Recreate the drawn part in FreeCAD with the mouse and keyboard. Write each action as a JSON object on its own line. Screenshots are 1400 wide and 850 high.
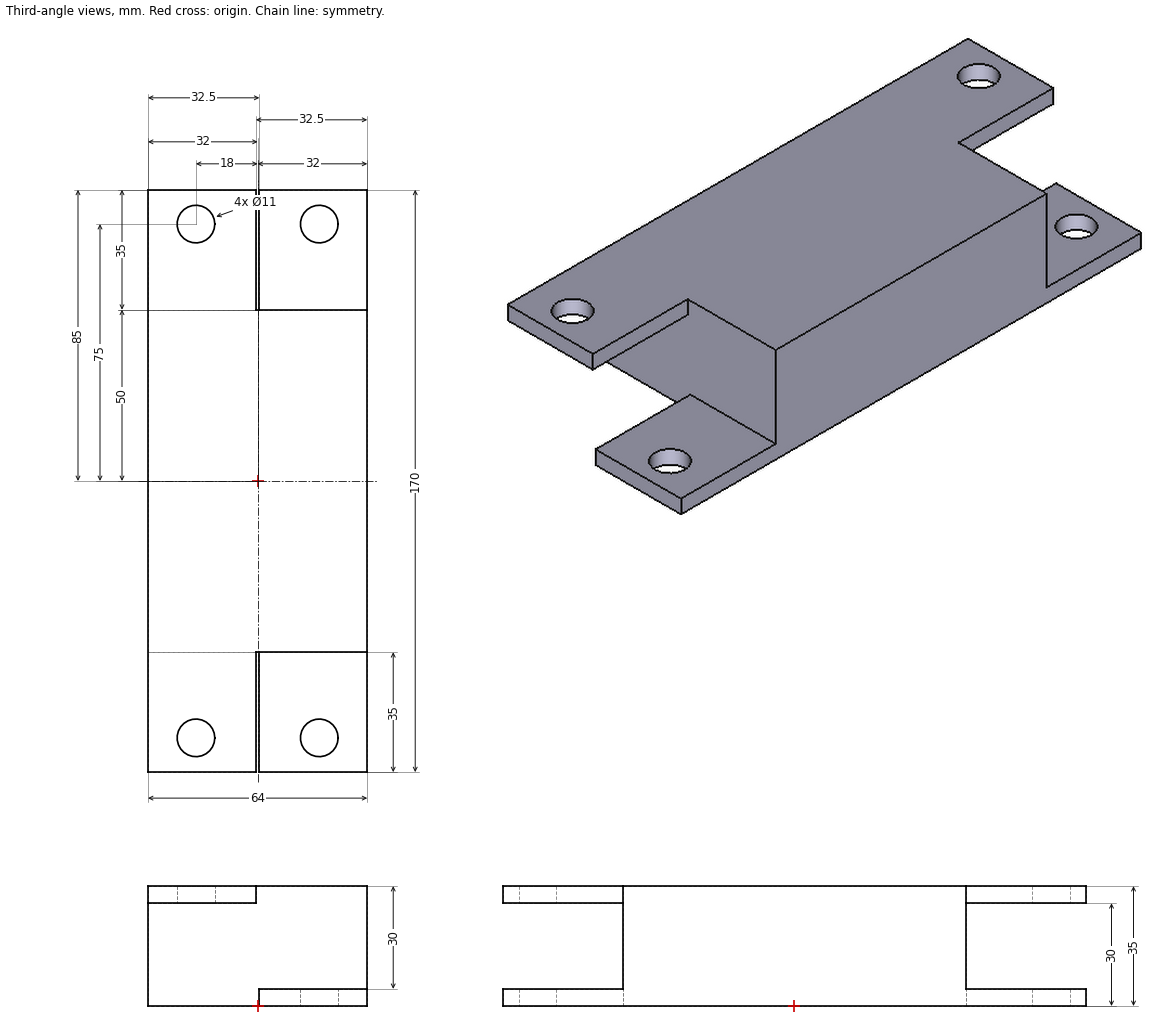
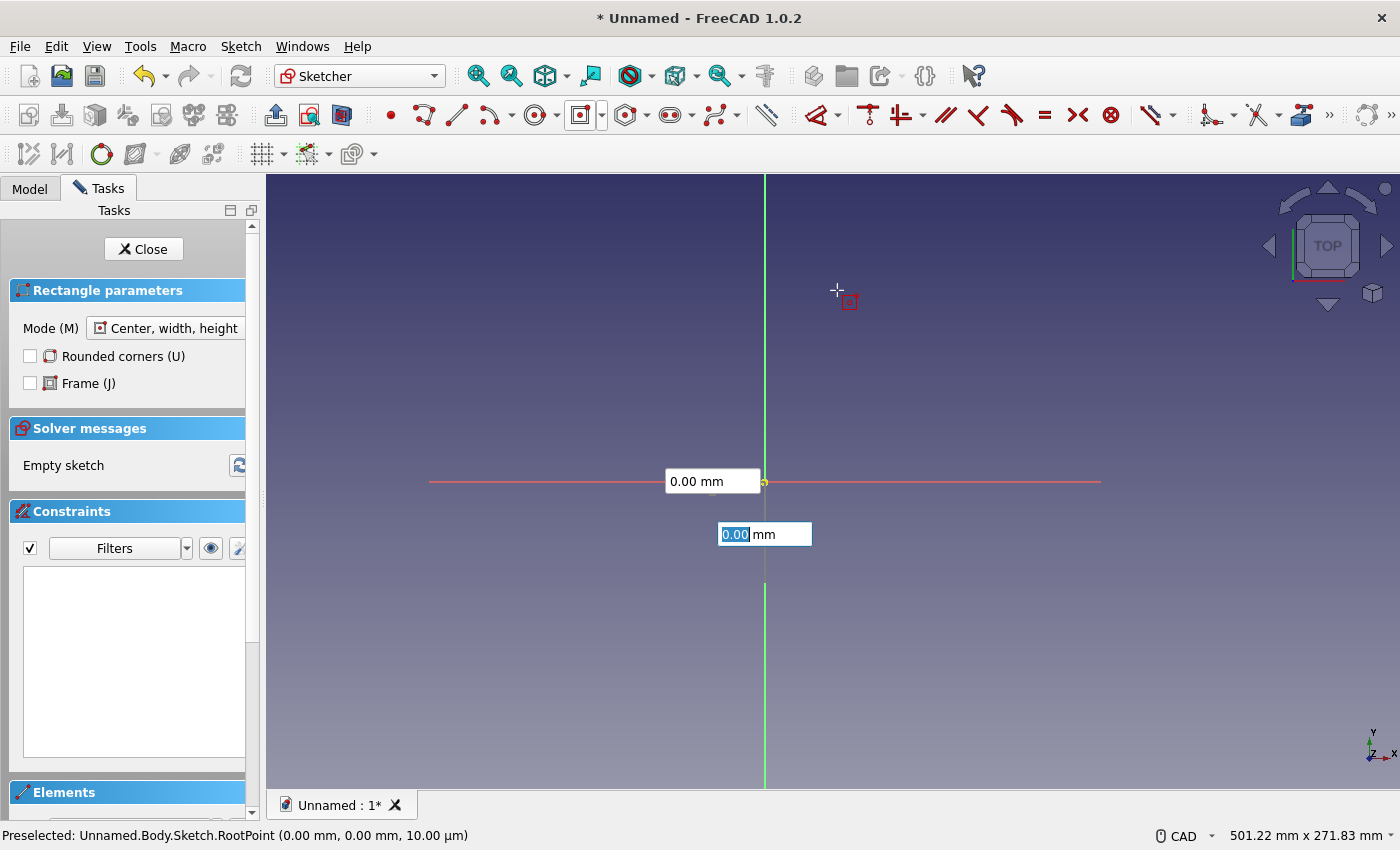
{"action": "type", "text": "64"}
{"action": "key", "text": "Tab"}
{"action": "type", "text": "170"}
{"action": "key", "text": "Return"}
{"action": "key", "text": "Escape"}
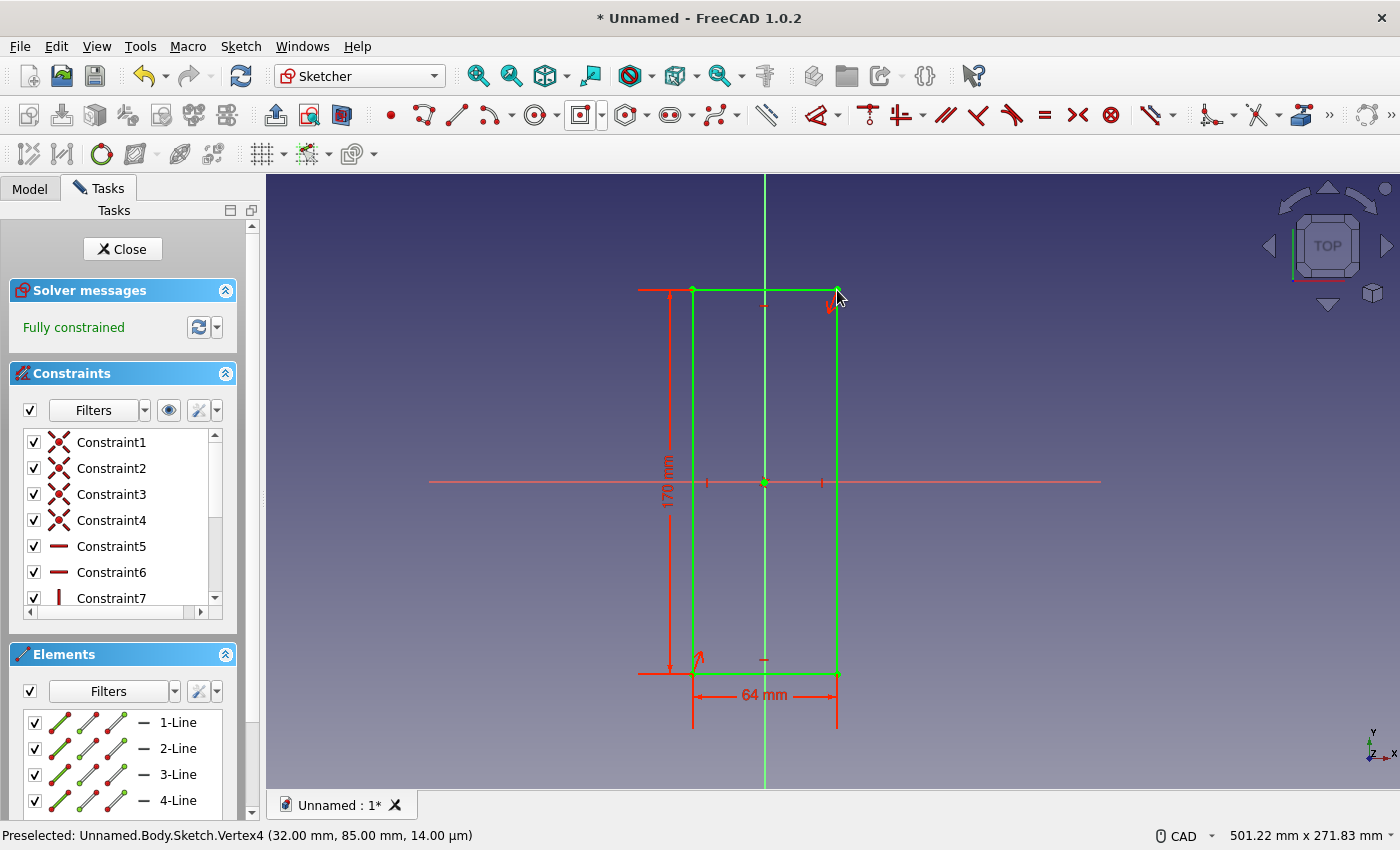
{"action": "left_click", "coordinate": [123, 249]}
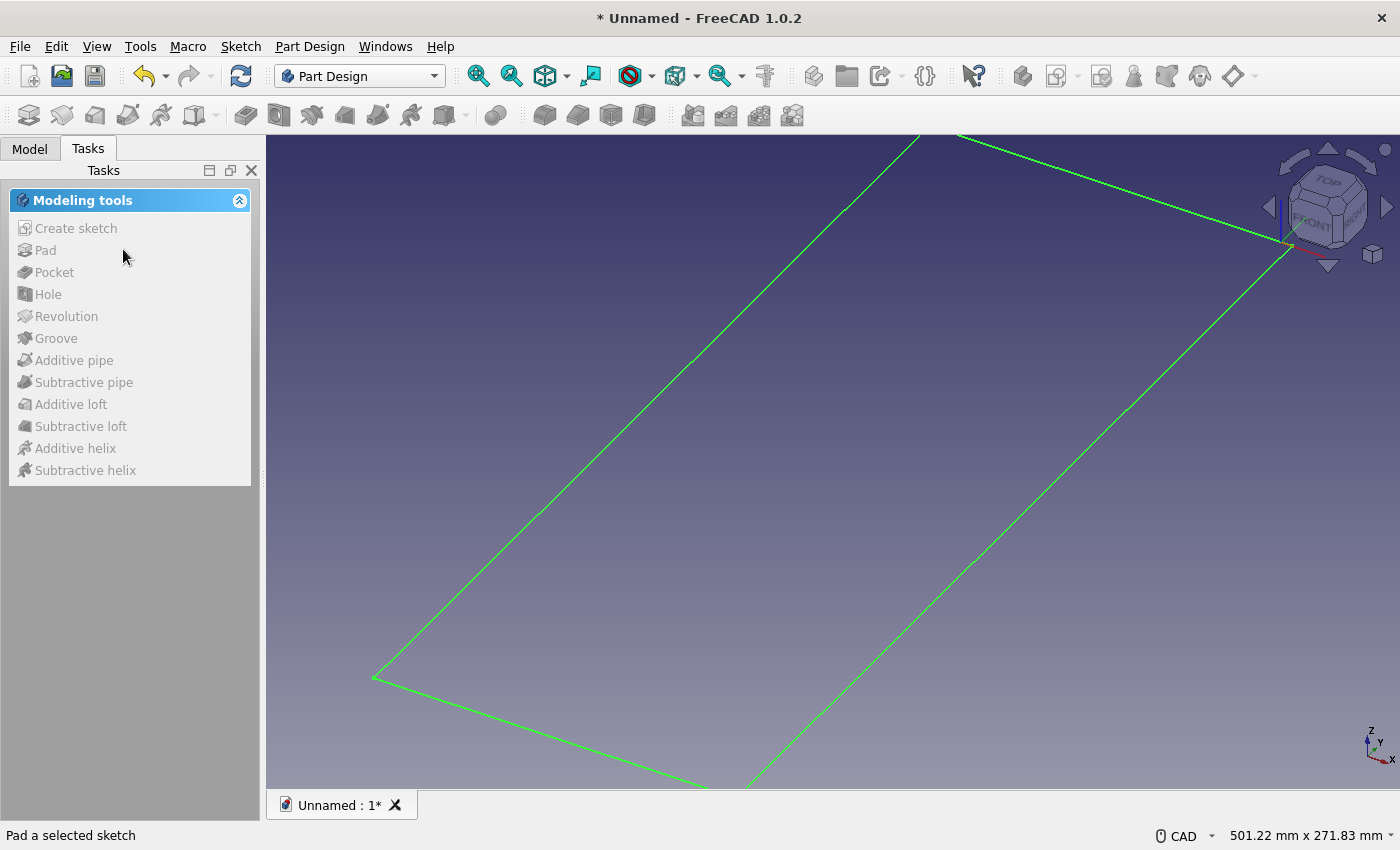
{"action": "left_click", "coordinate": [29, 116]}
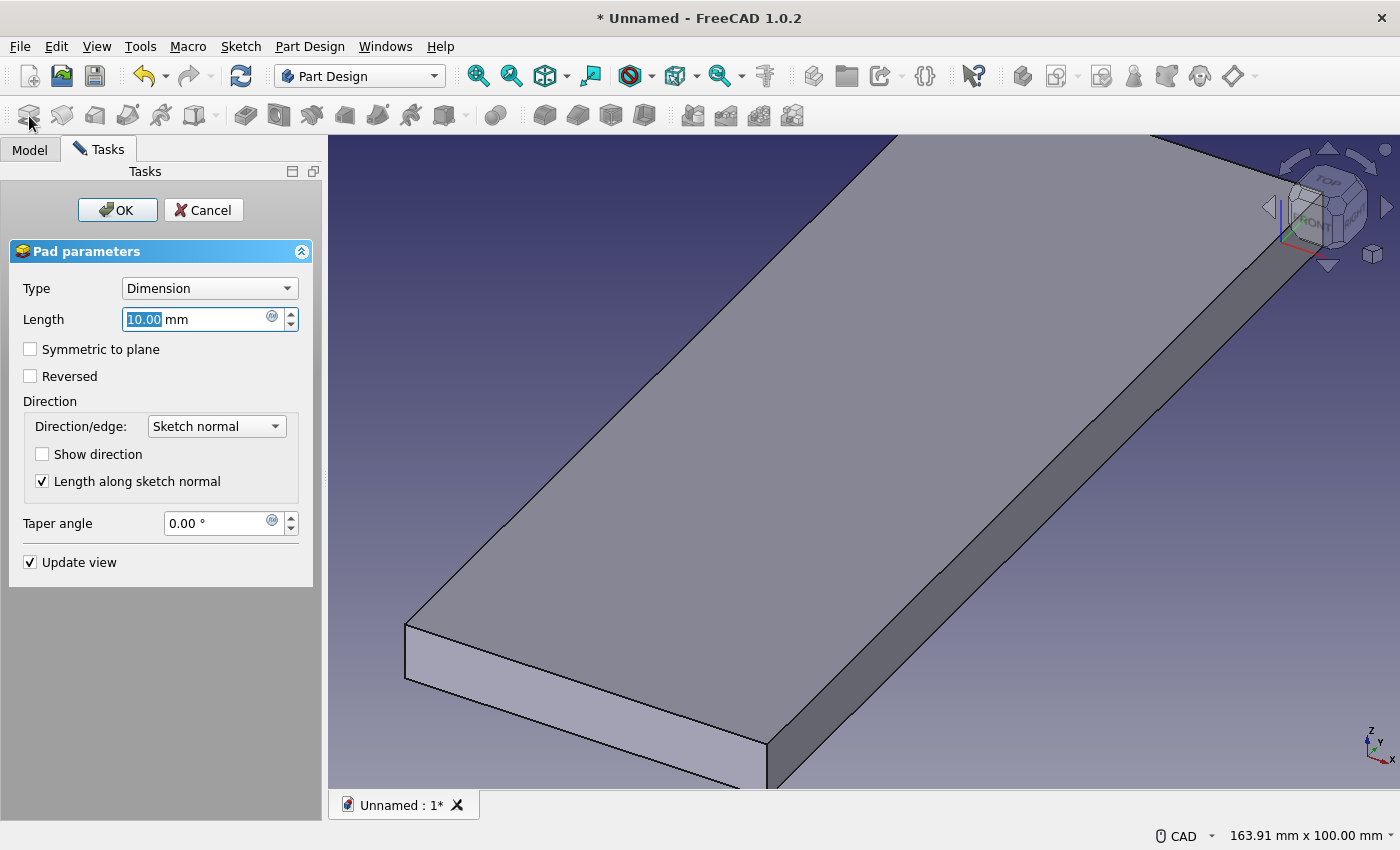
{"action": "type", "text": "35"}
{"action": "key", "text": "Tab"}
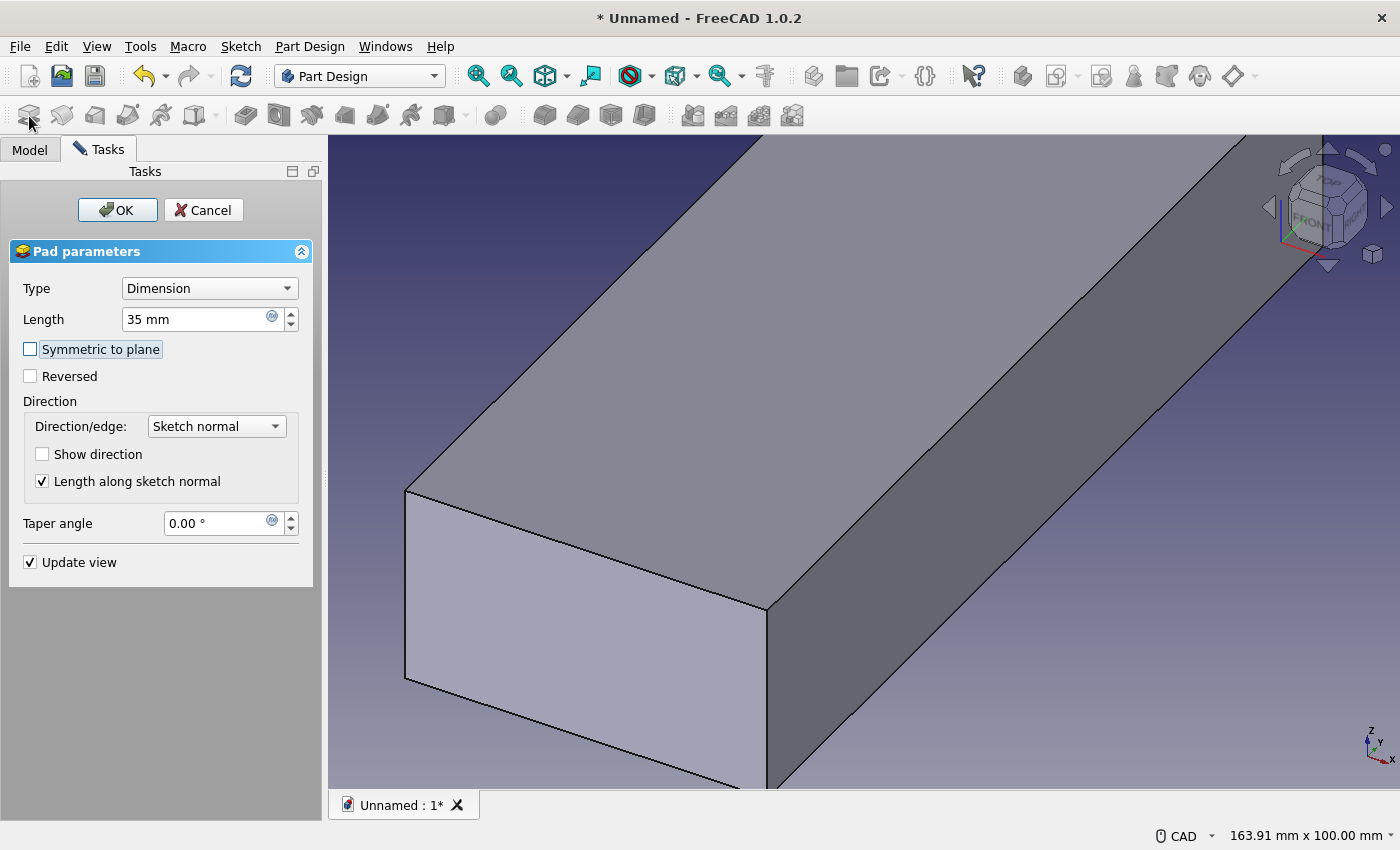
{"action": "left_click", "coordinate": [118, 210]}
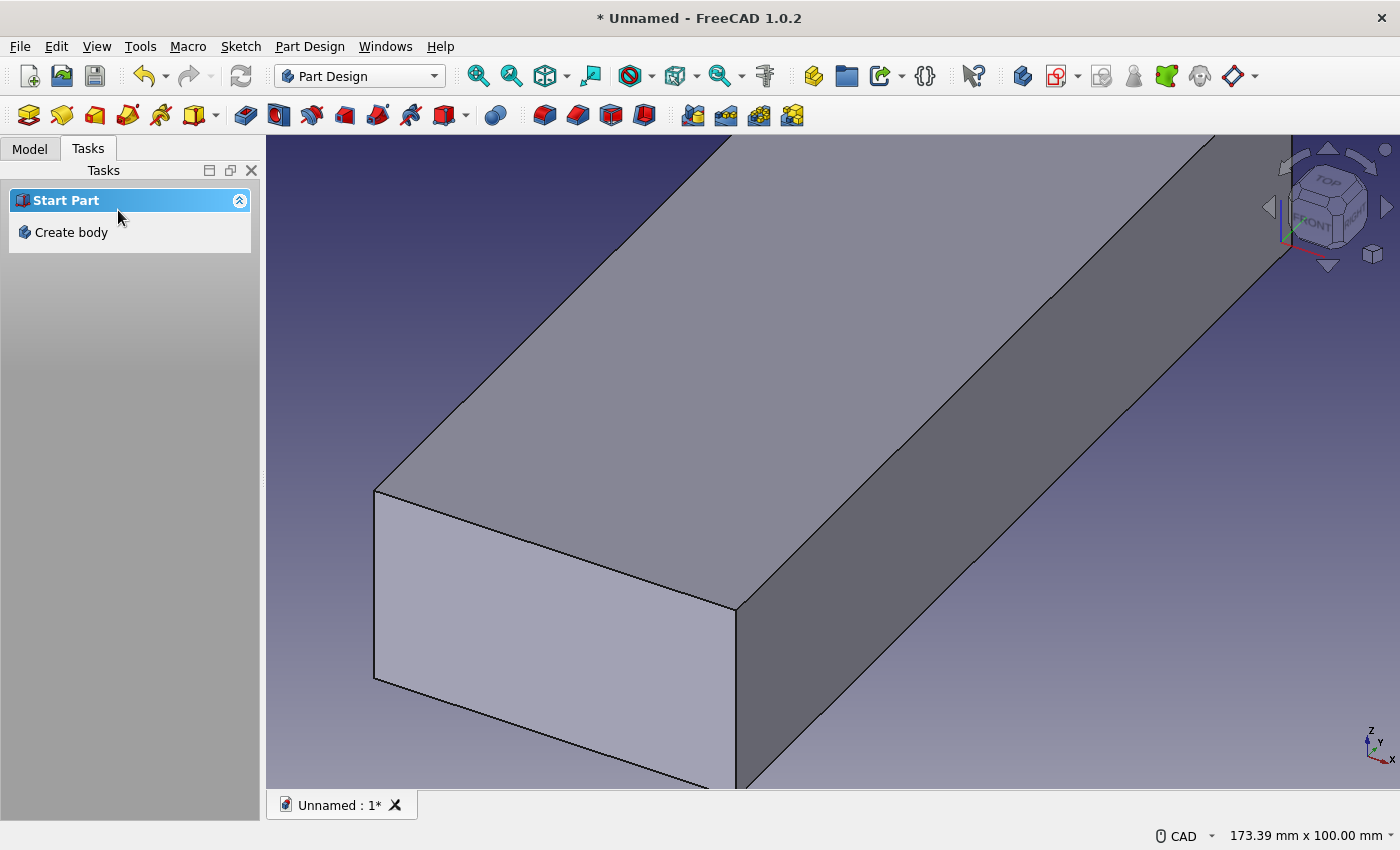
{"action": "left_click", "coordinate": [479, 76]}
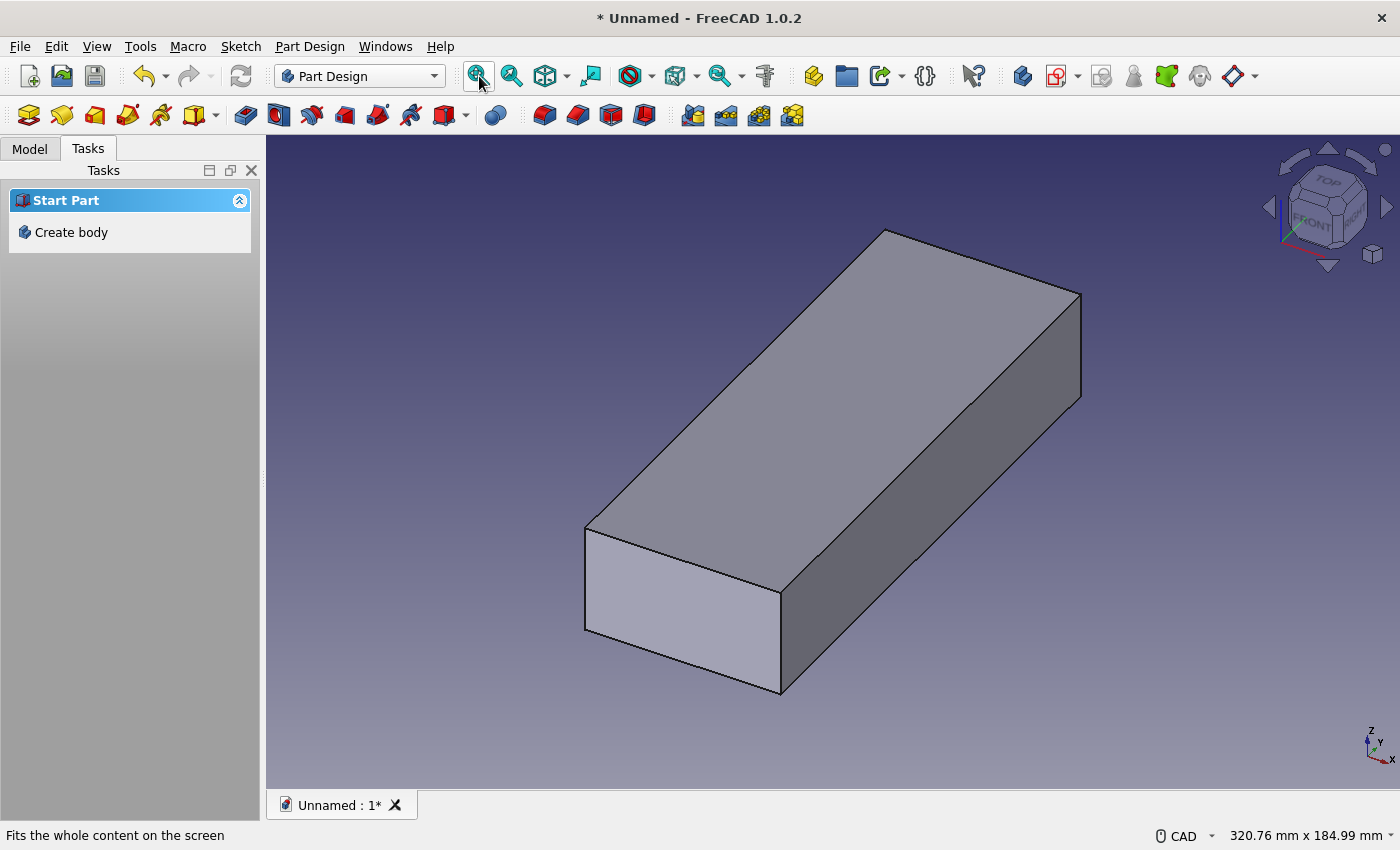
{"action": "left_click", "coordinate": [919, 325]}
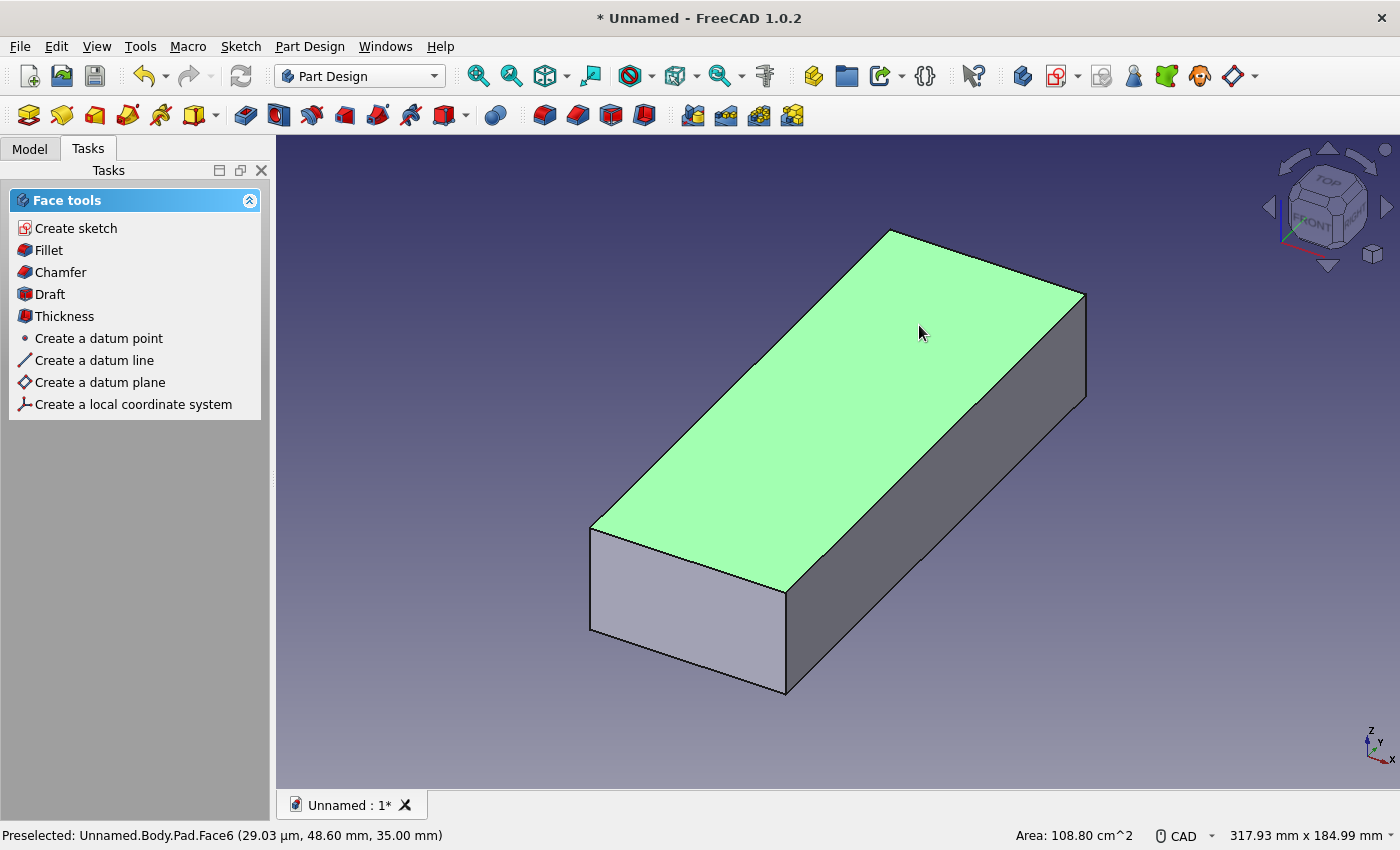
{"action": "left_click", "coordinate": [1056, 76]}